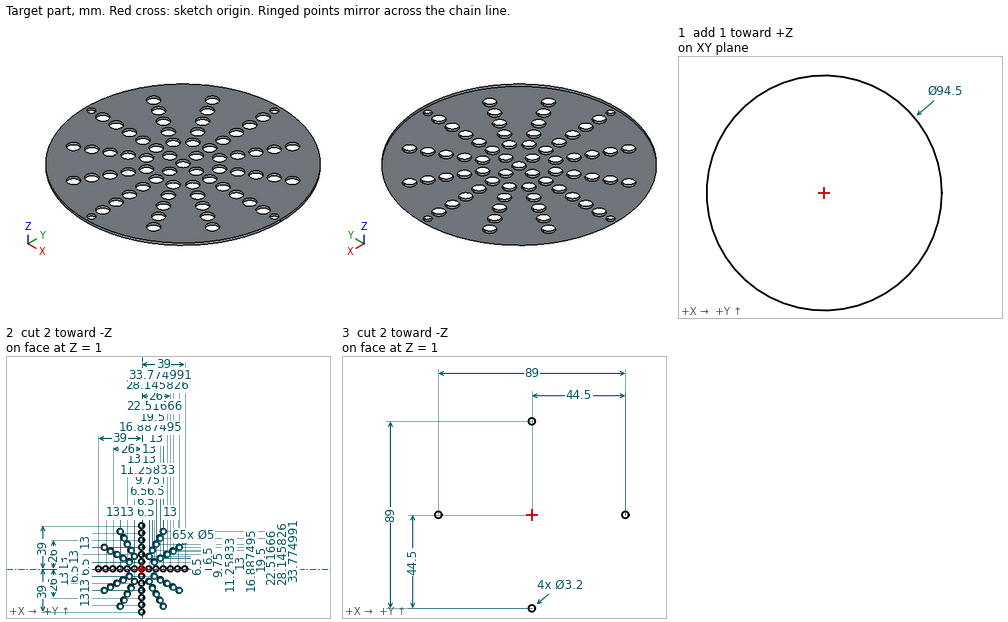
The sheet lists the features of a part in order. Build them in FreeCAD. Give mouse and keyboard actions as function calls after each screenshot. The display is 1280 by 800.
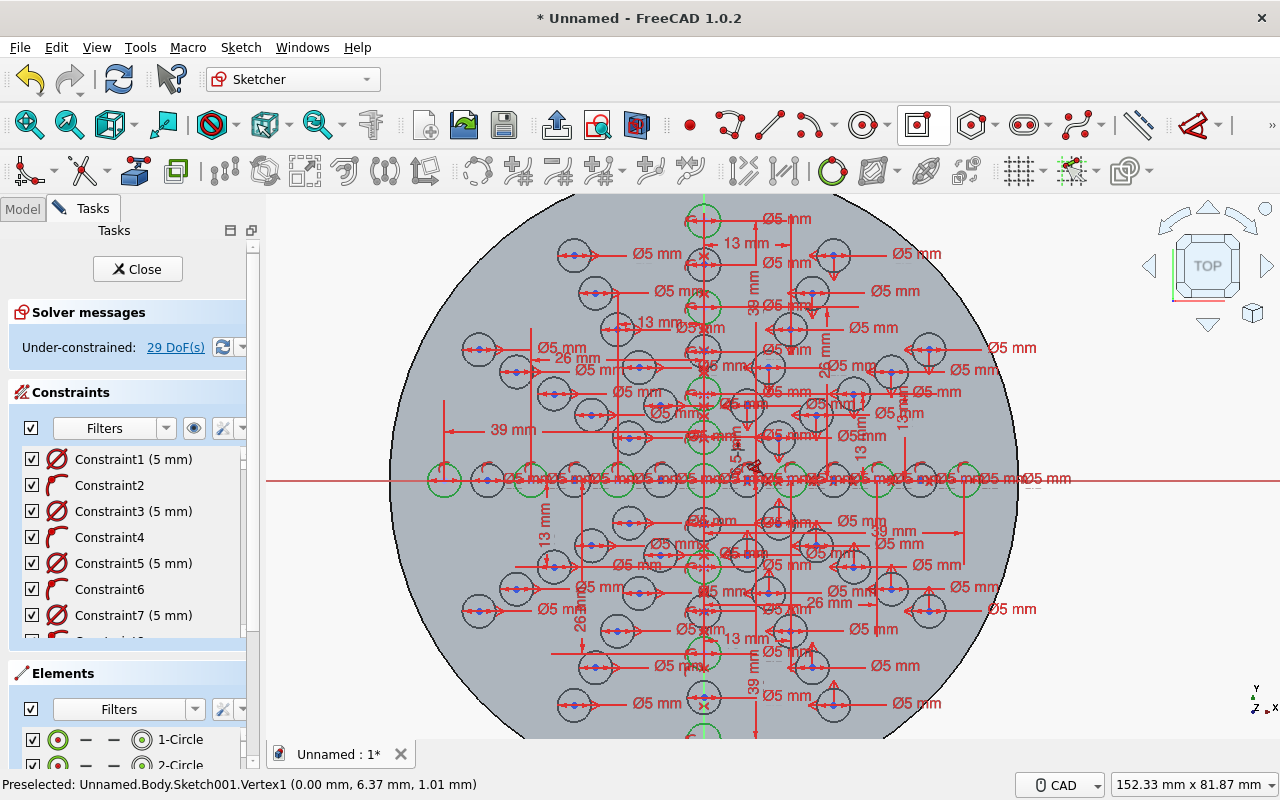
click(747, 406)
click(736, 372)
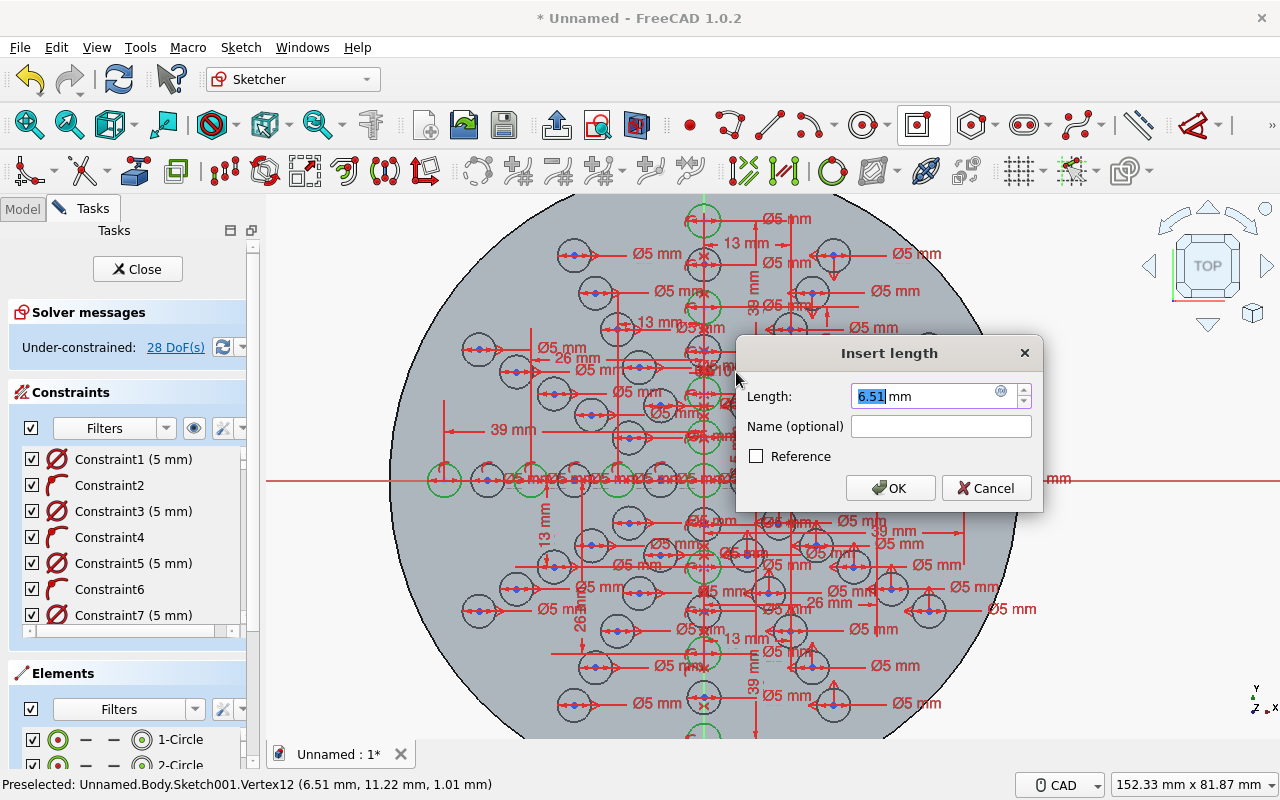
text(6.5)
key(Return)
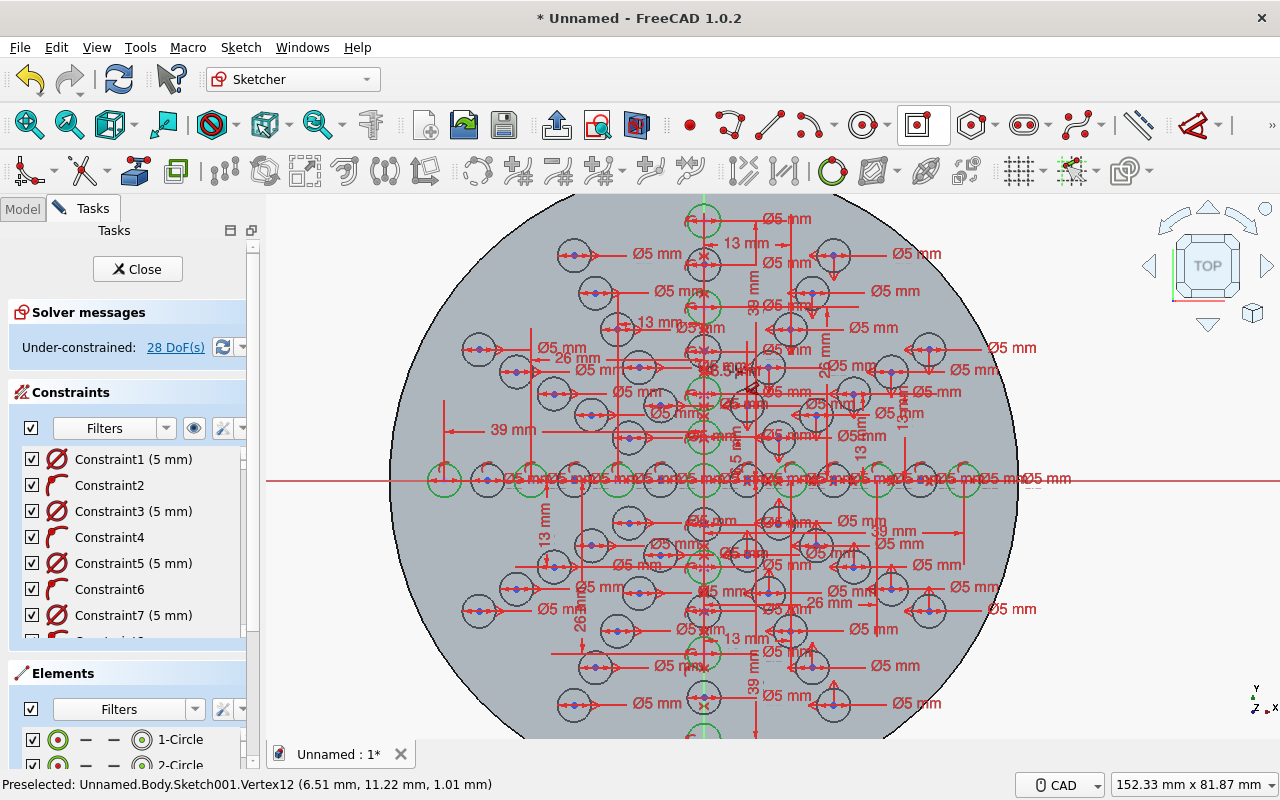
click(779, 438)
click(813, 459)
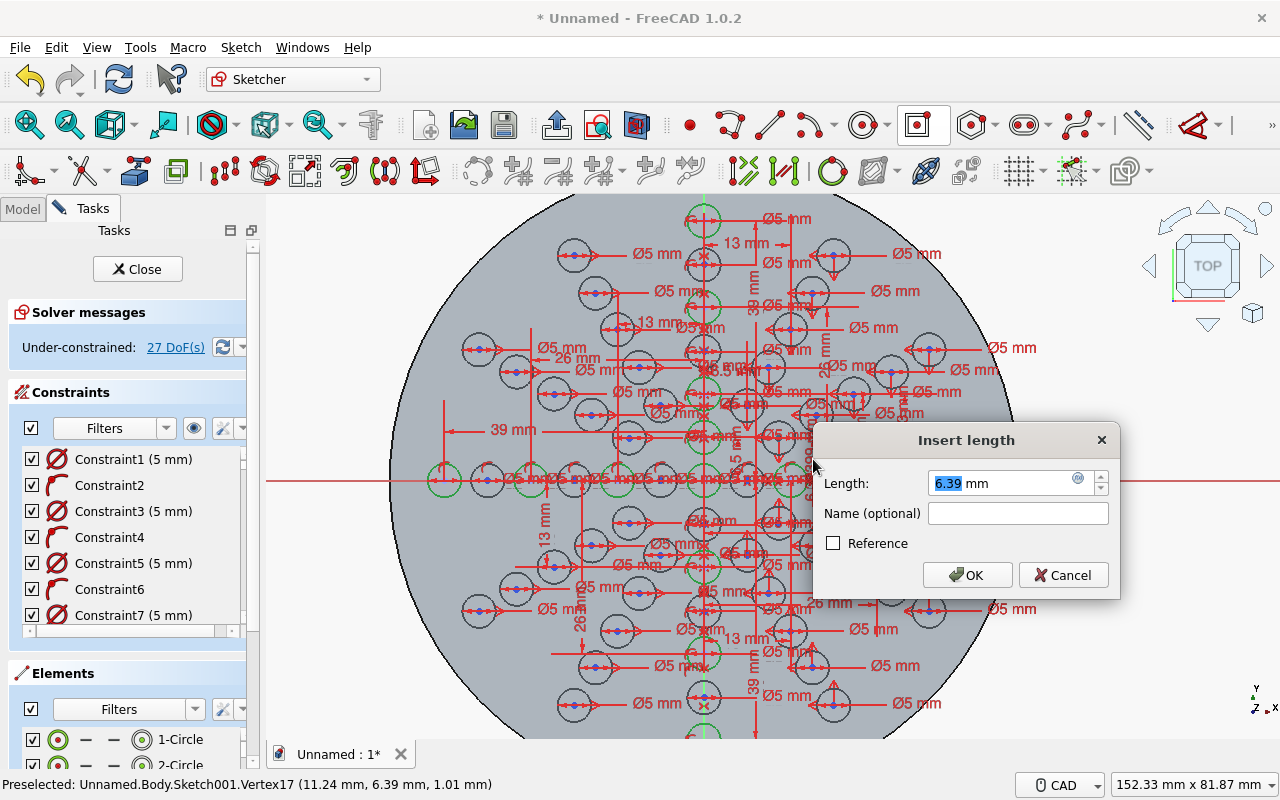
text(6.5)
key(Return)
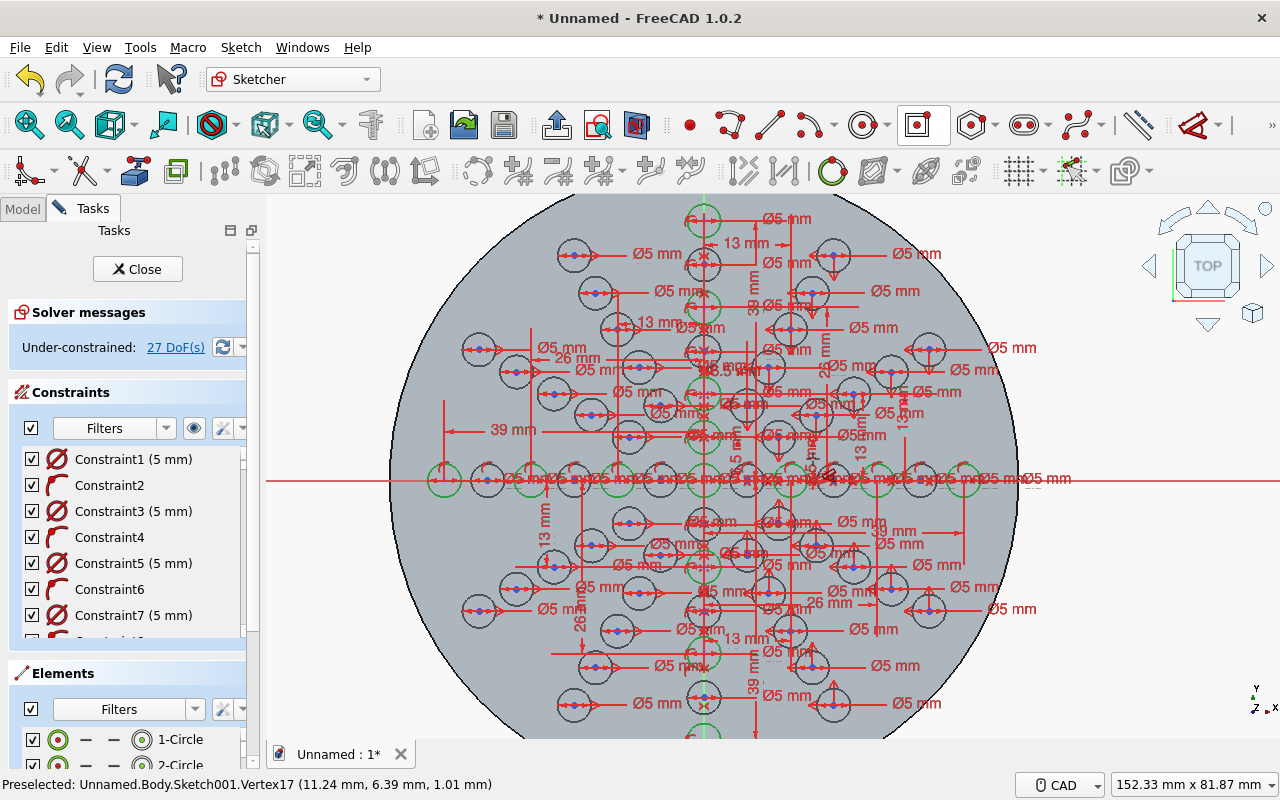
click(747, 481)
click(735, 515)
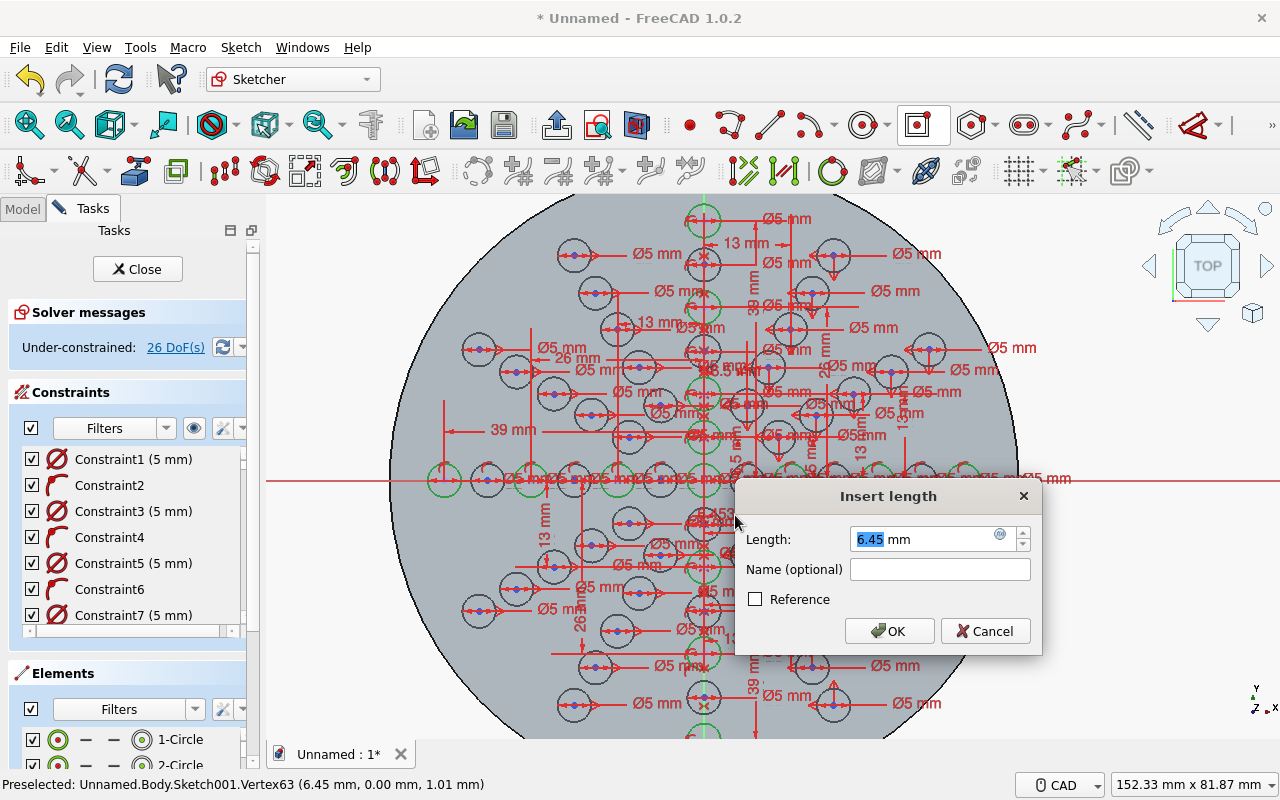
text(6.5)
key(Return)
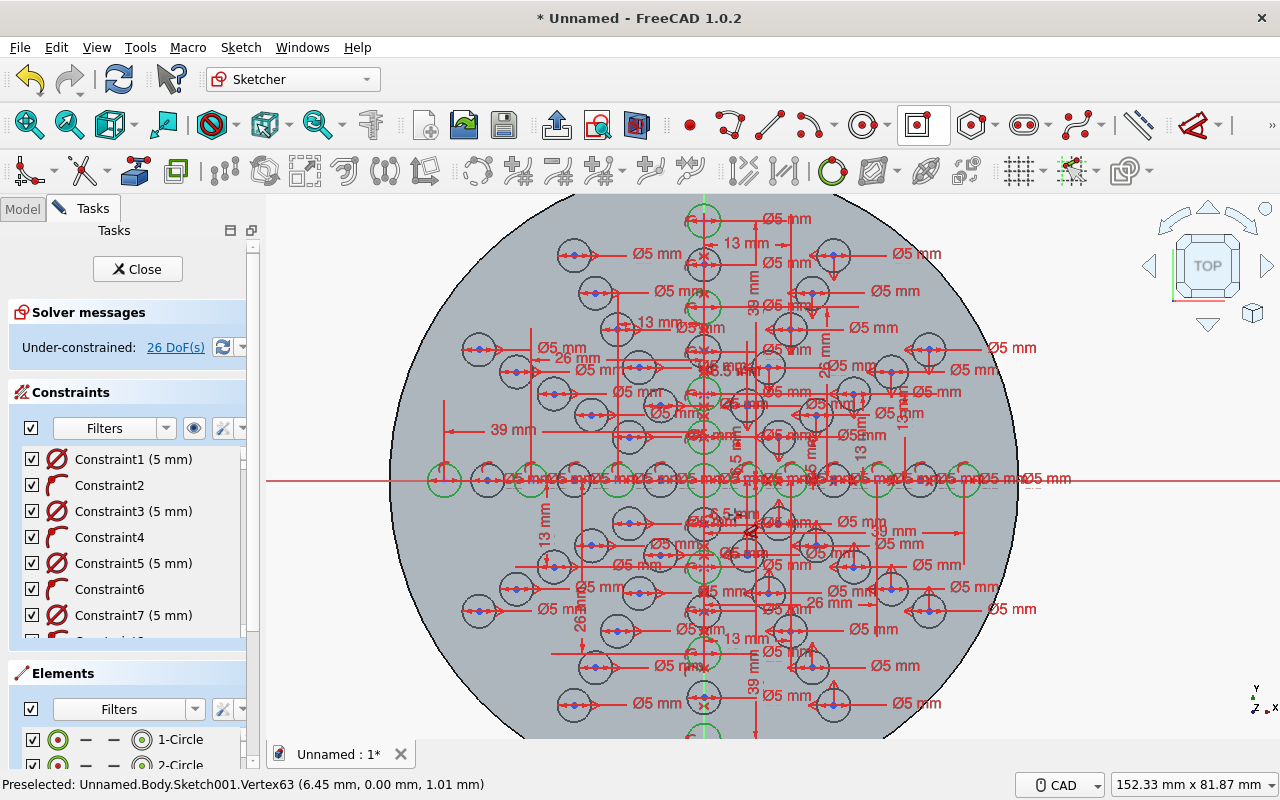
click(704, 525)
click(810, 513)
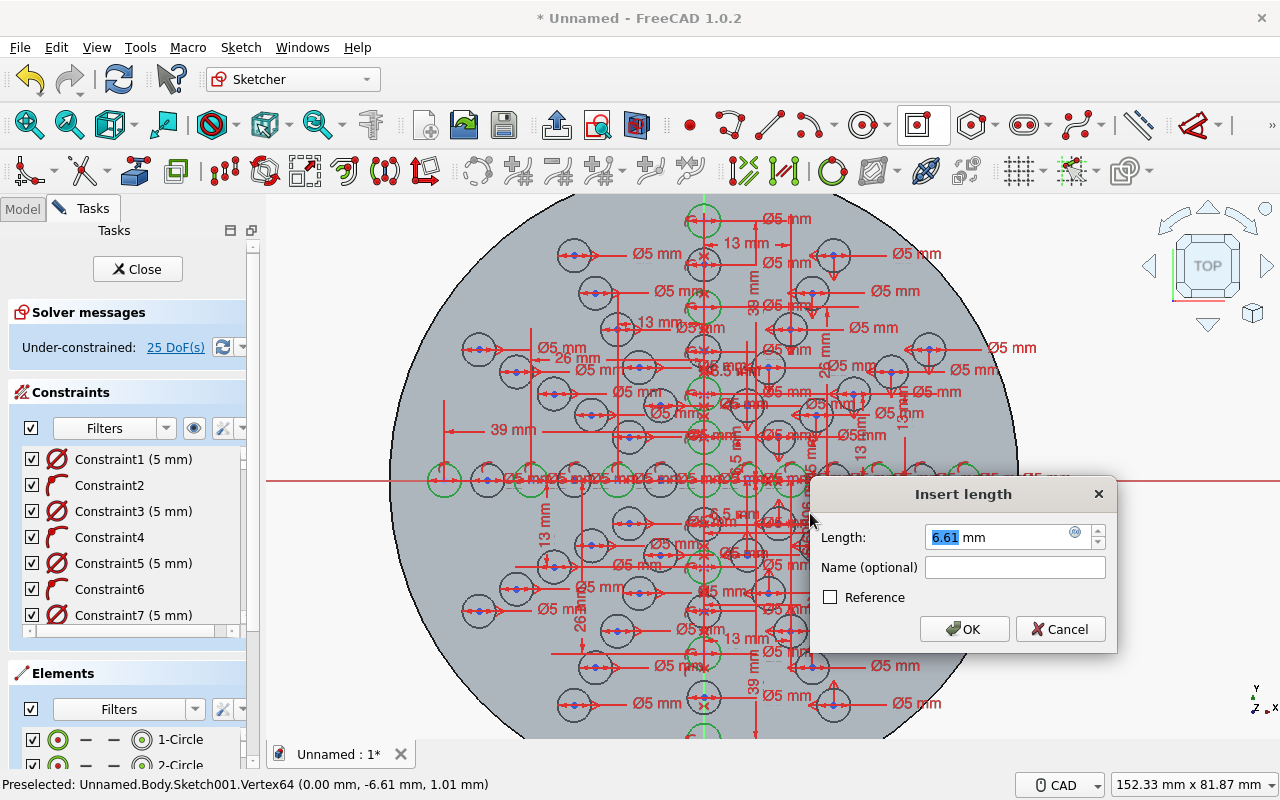
text(6.5)
key(Return)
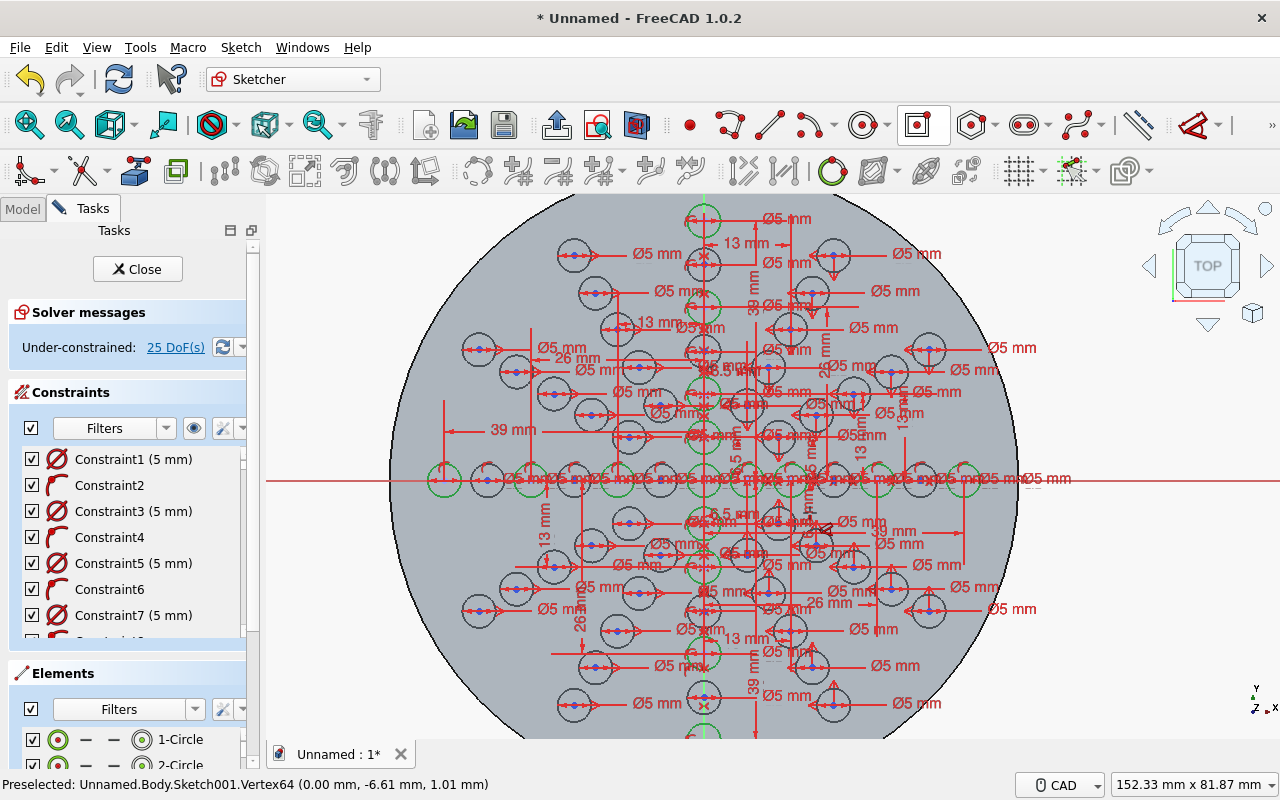
click(661, 481)
click(667, 447)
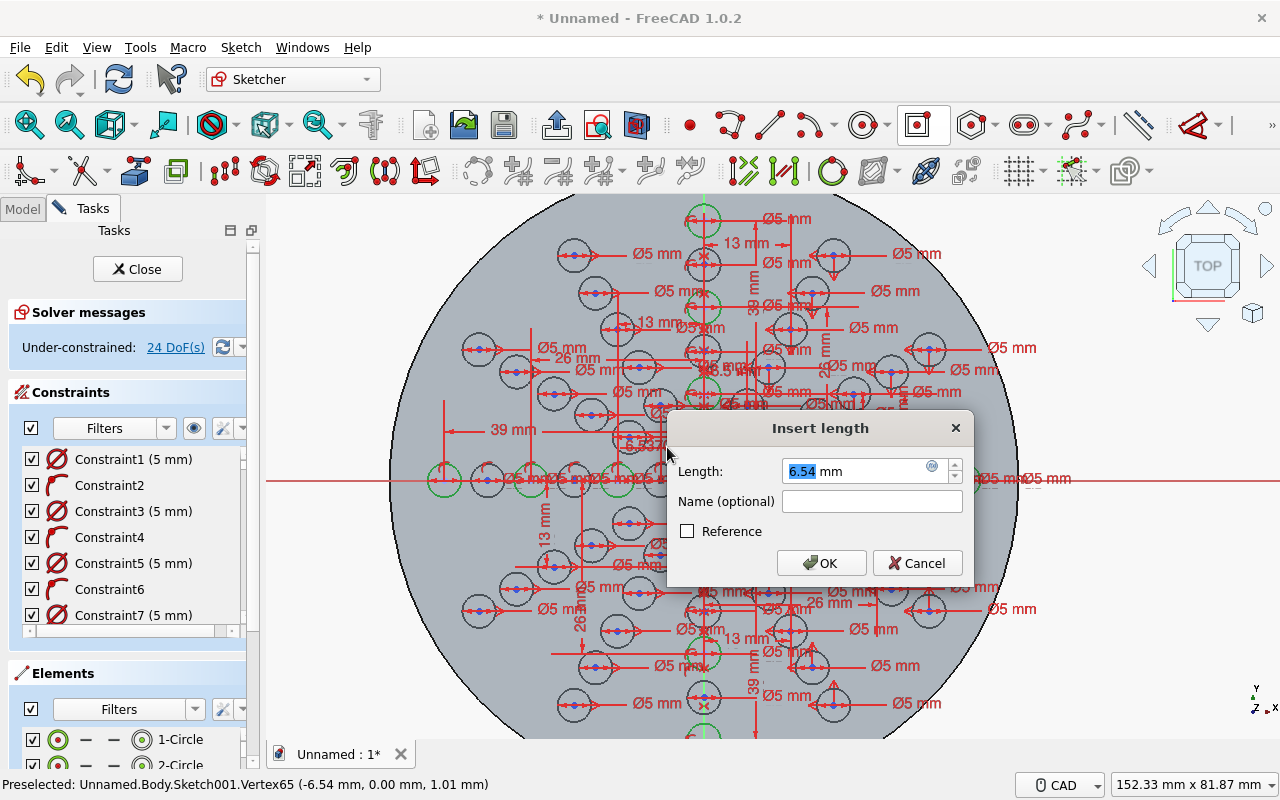
text(6.5)
key(Return)